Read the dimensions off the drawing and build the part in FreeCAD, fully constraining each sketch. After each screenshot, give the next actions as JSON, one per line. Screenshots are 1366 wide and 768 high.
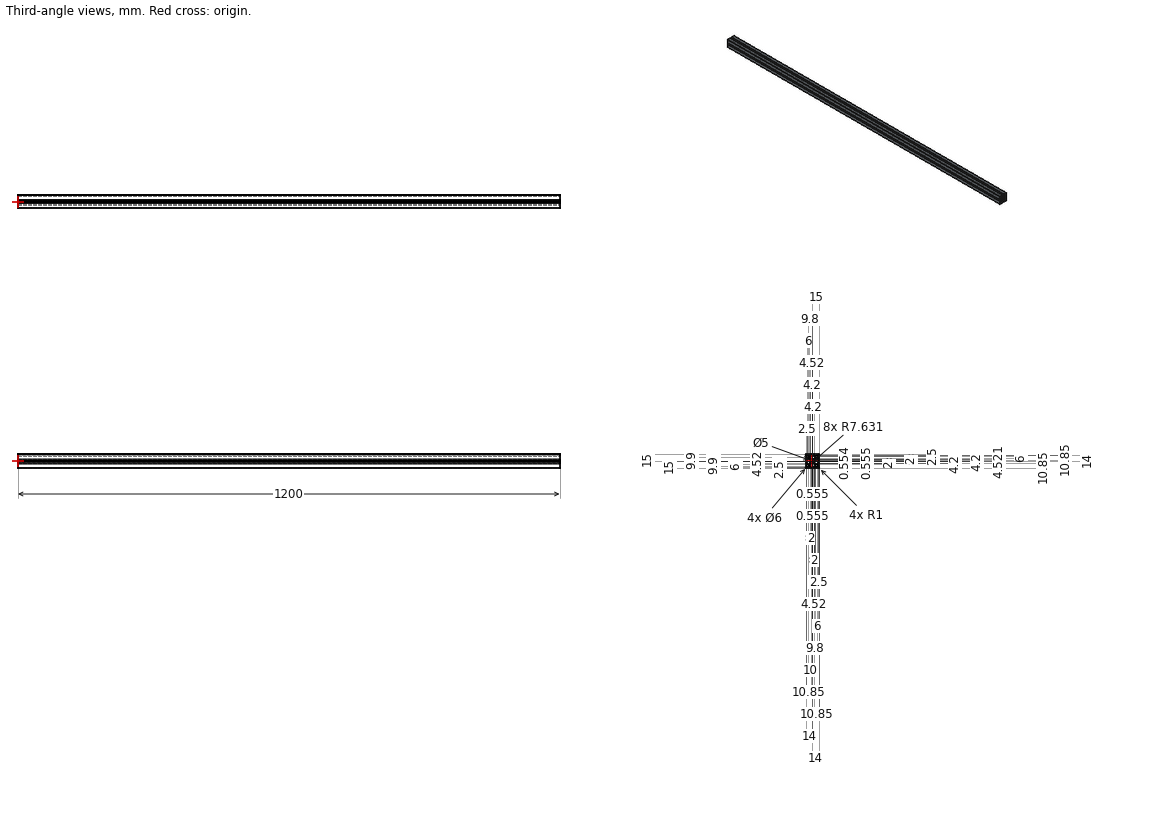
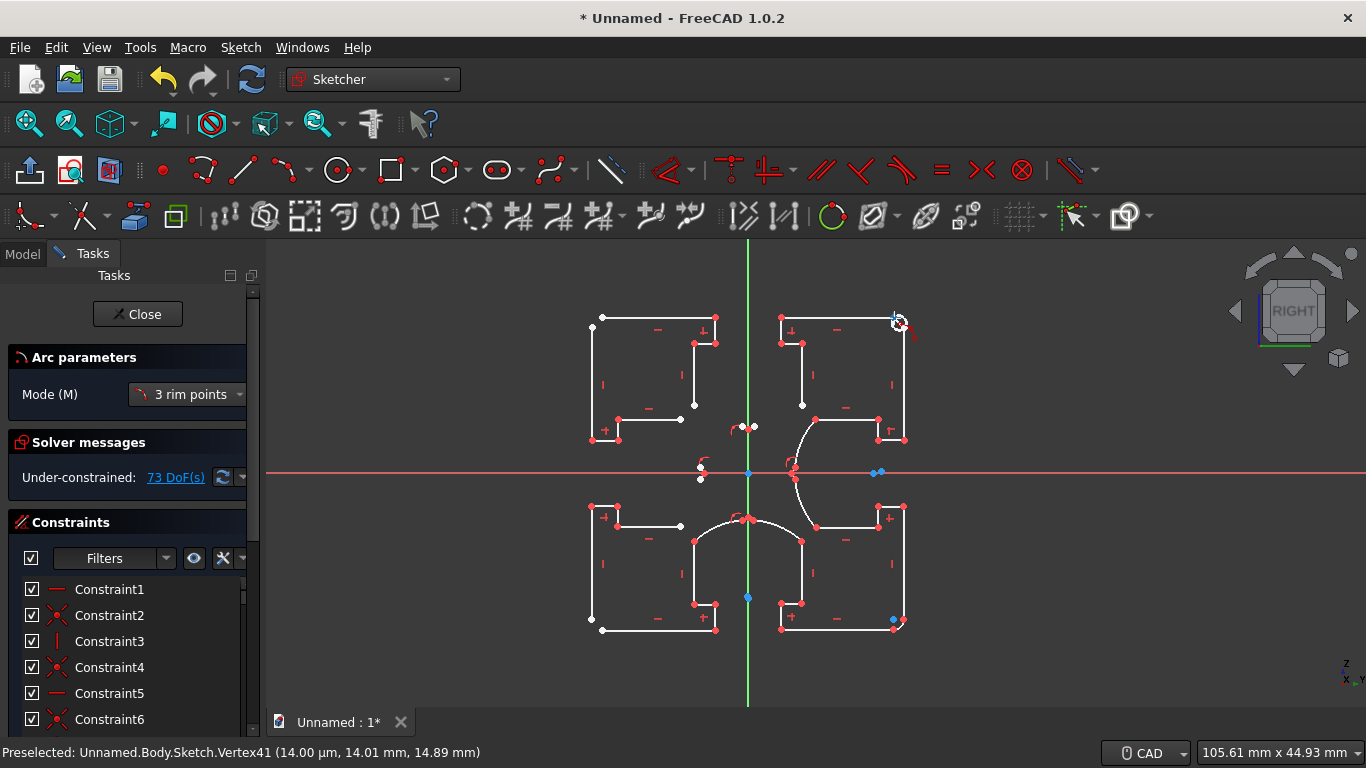
{"action": "scroll", "coordinate": [901, 320], "scroll_direction": "up", "scroll_amount": 9}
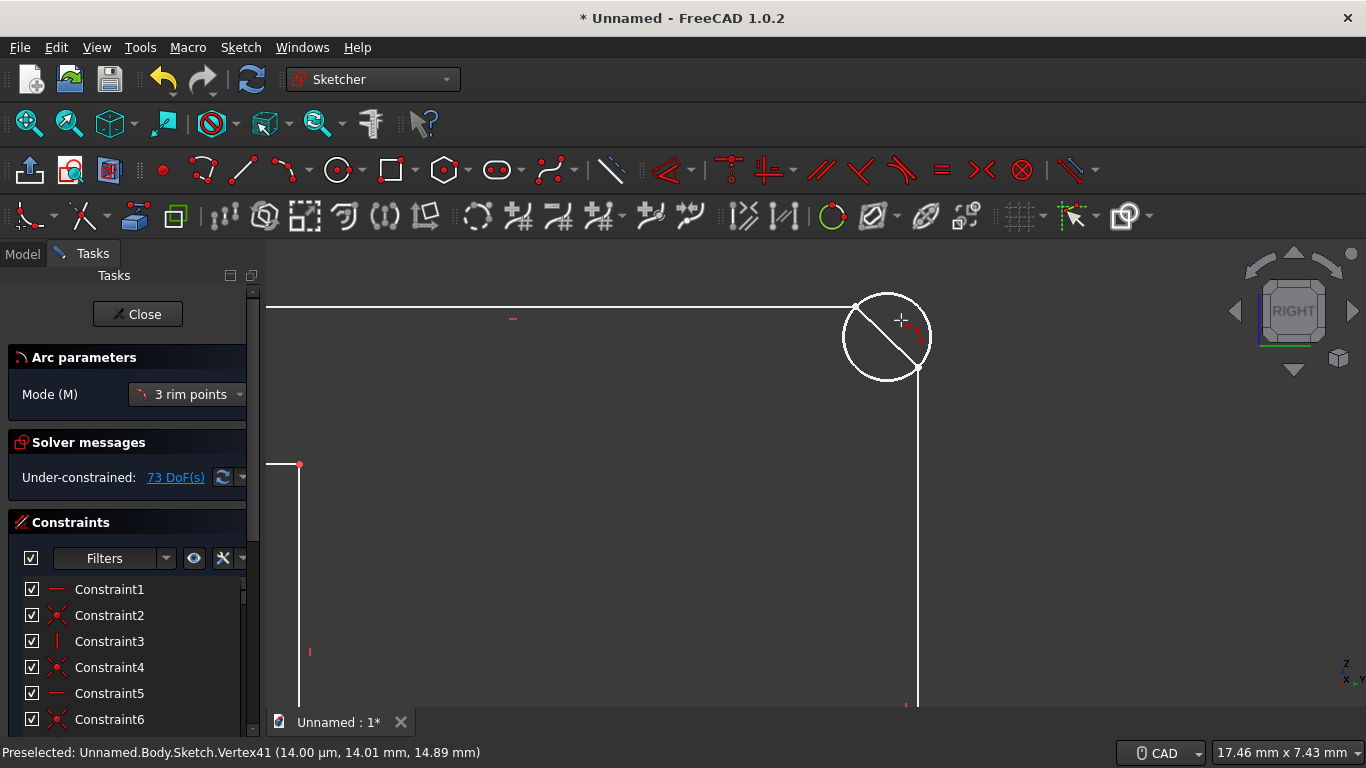
{"action": "left_click", "coordinate": [900, 318]}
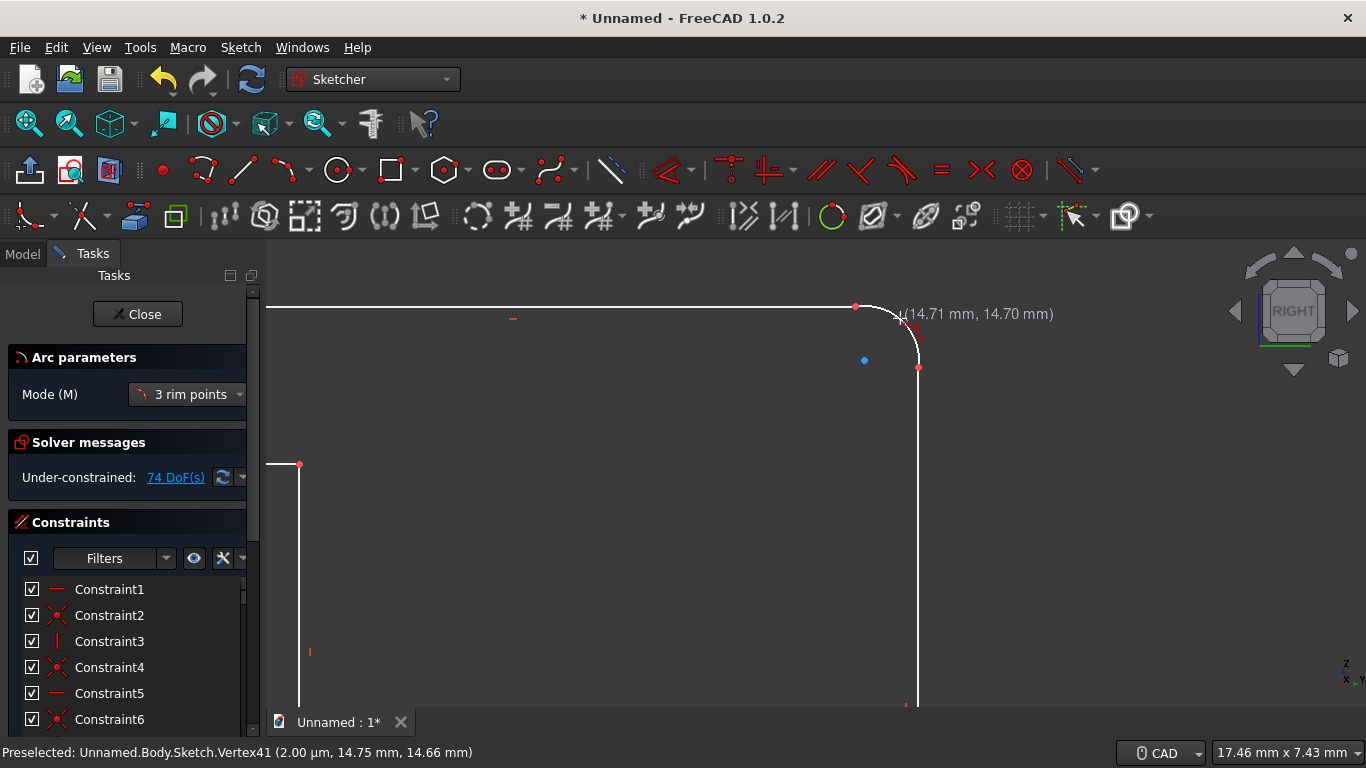
{"action": "scroll", "coordinate": [901, 320], "scroll_direction": "down", "scroll_amount": 9}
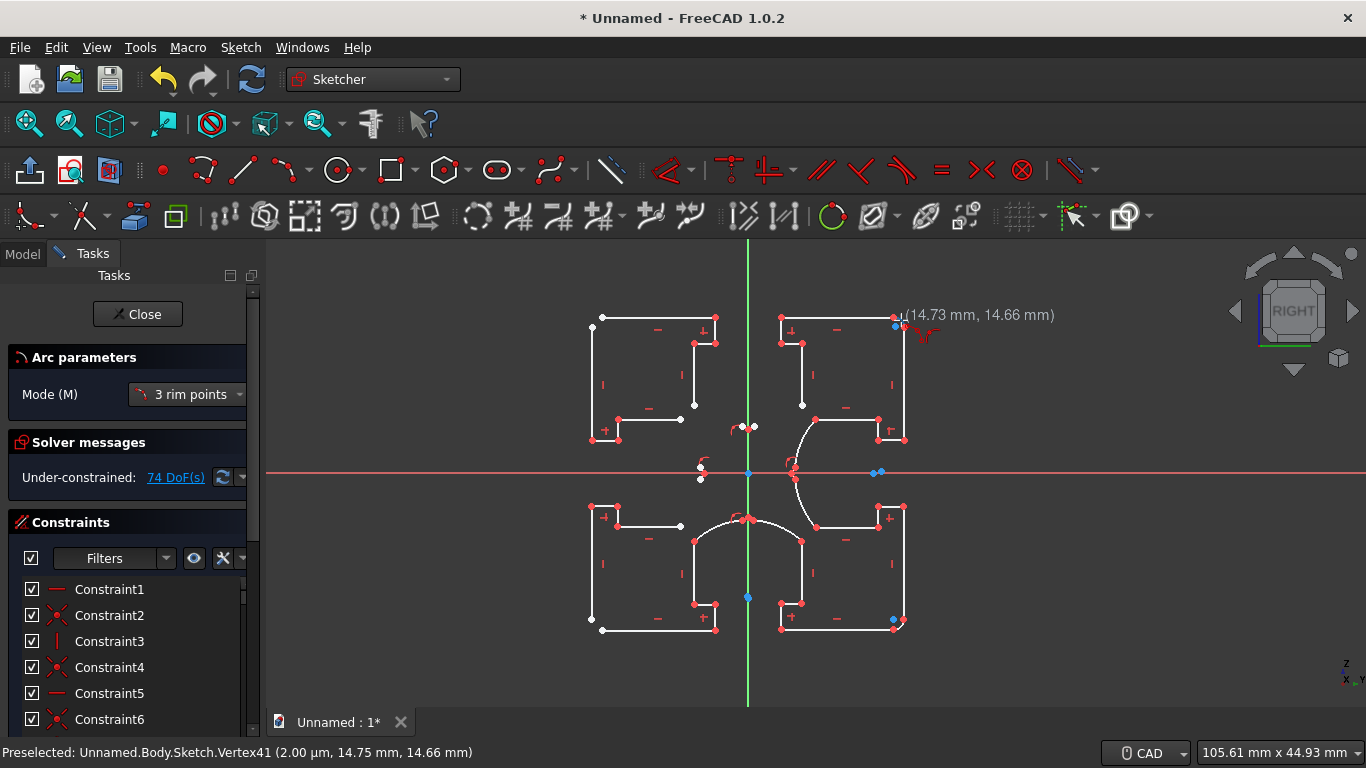
{"action": "left_click", "coordinate": [802, 406]}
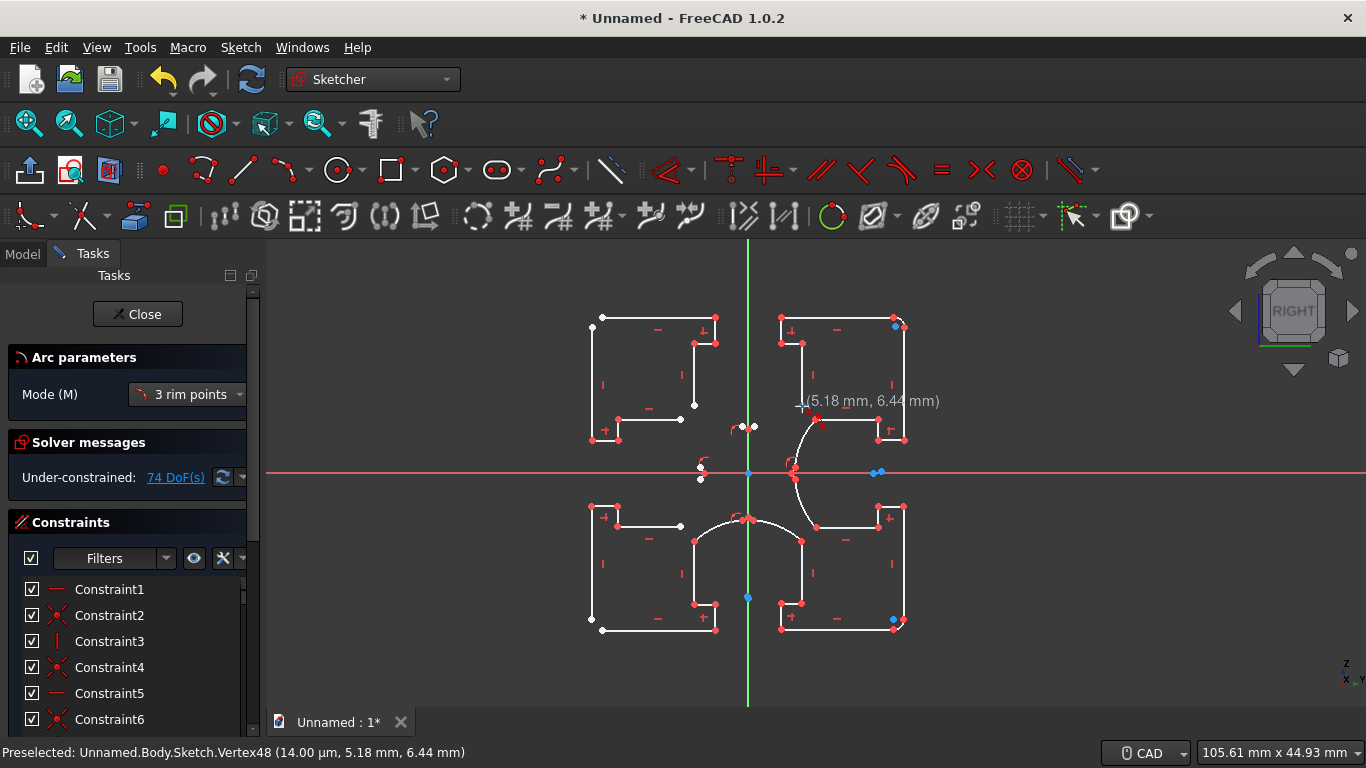
{"action": "scroll", "coordinate": [754, 426], "scroll_direction": "up", "scroll_amount": 8}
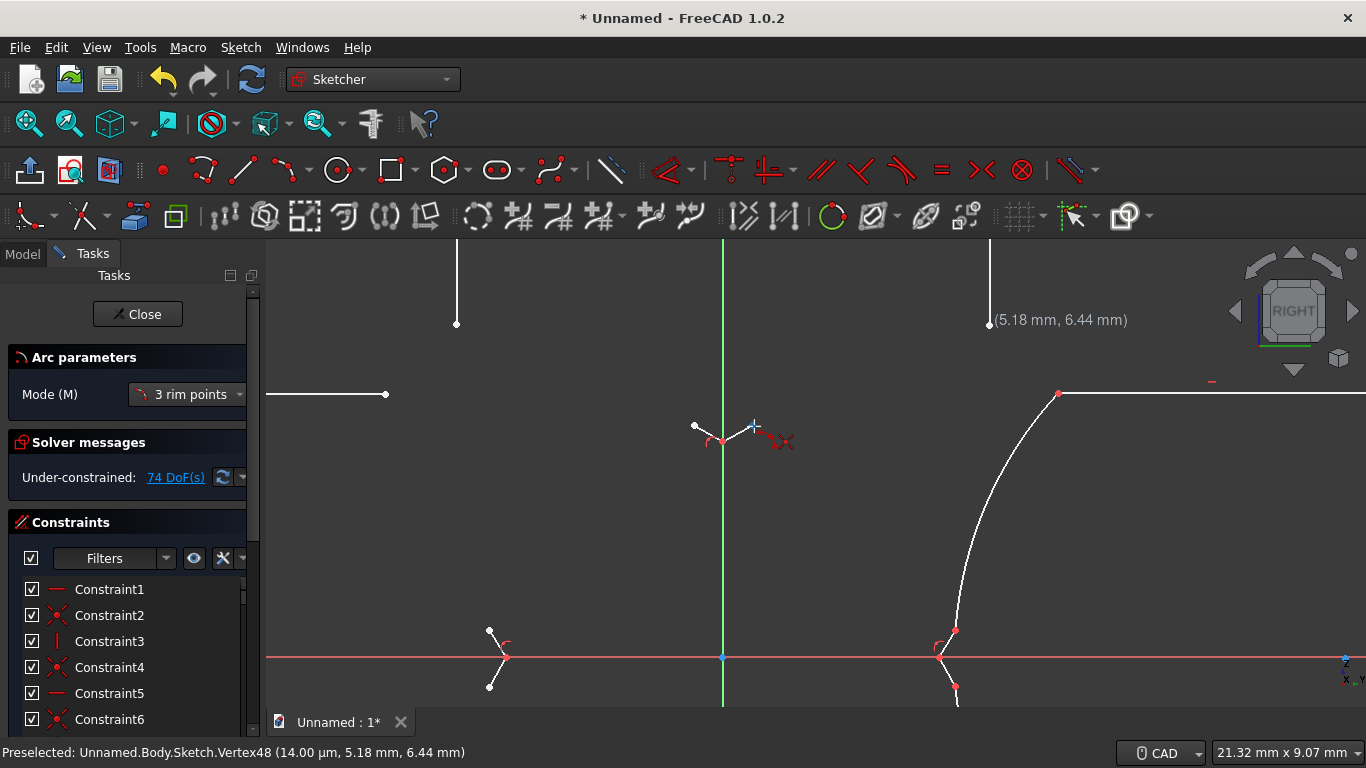
{"action": "left_click", "coordinate": [752, 426]}
{"action": "left_click", "coordinate": [879, 393]}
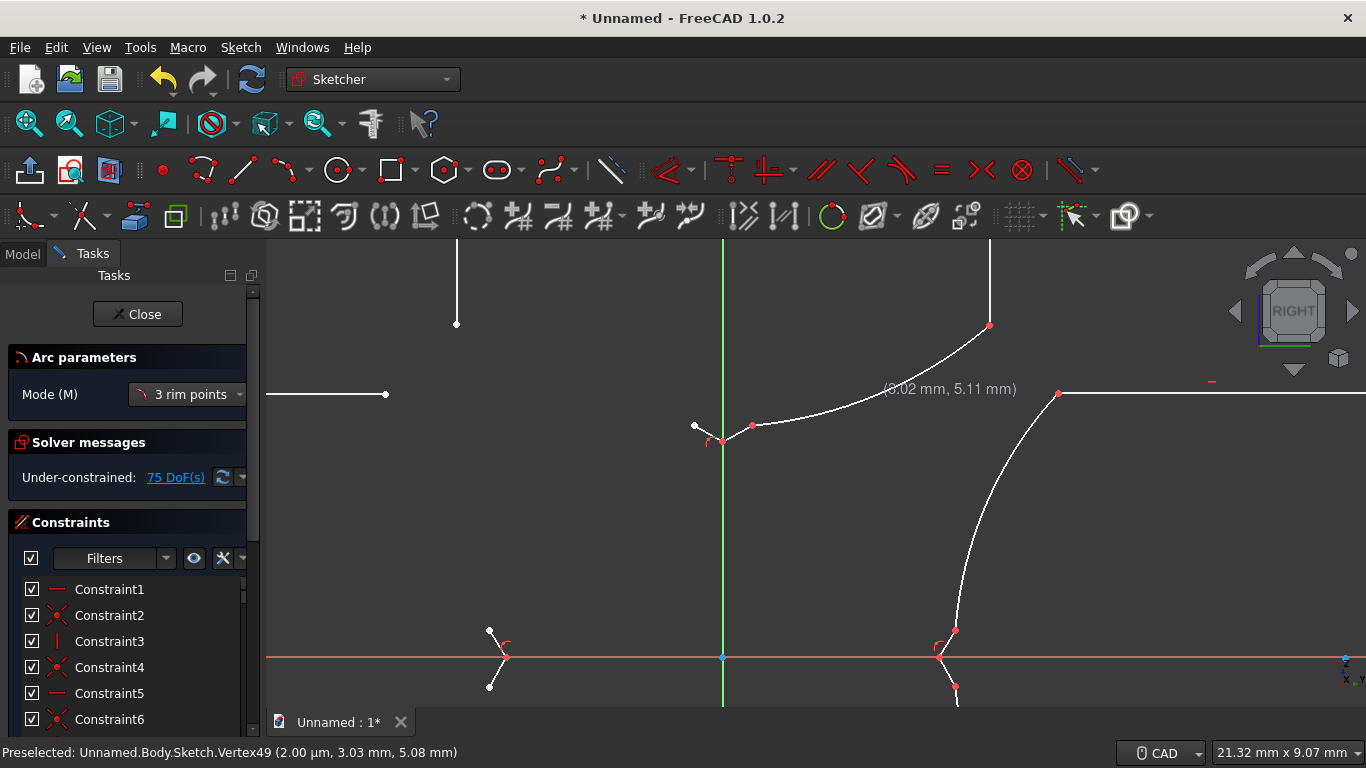
{"action": "left_click", "coordinate": [694, 426]}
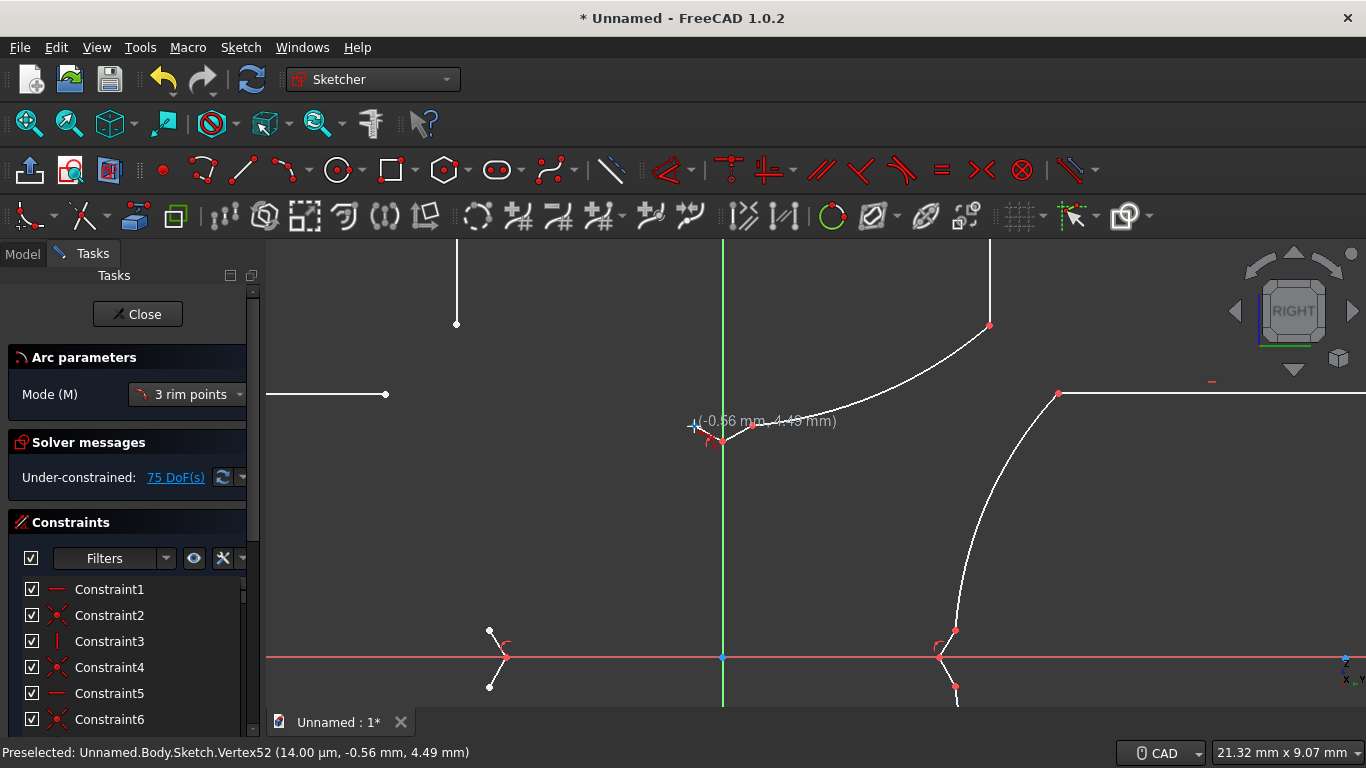
{"action": "scroll", "coordinate": [754, 426], "scroll_direction": "down", "scroll_amount": 8}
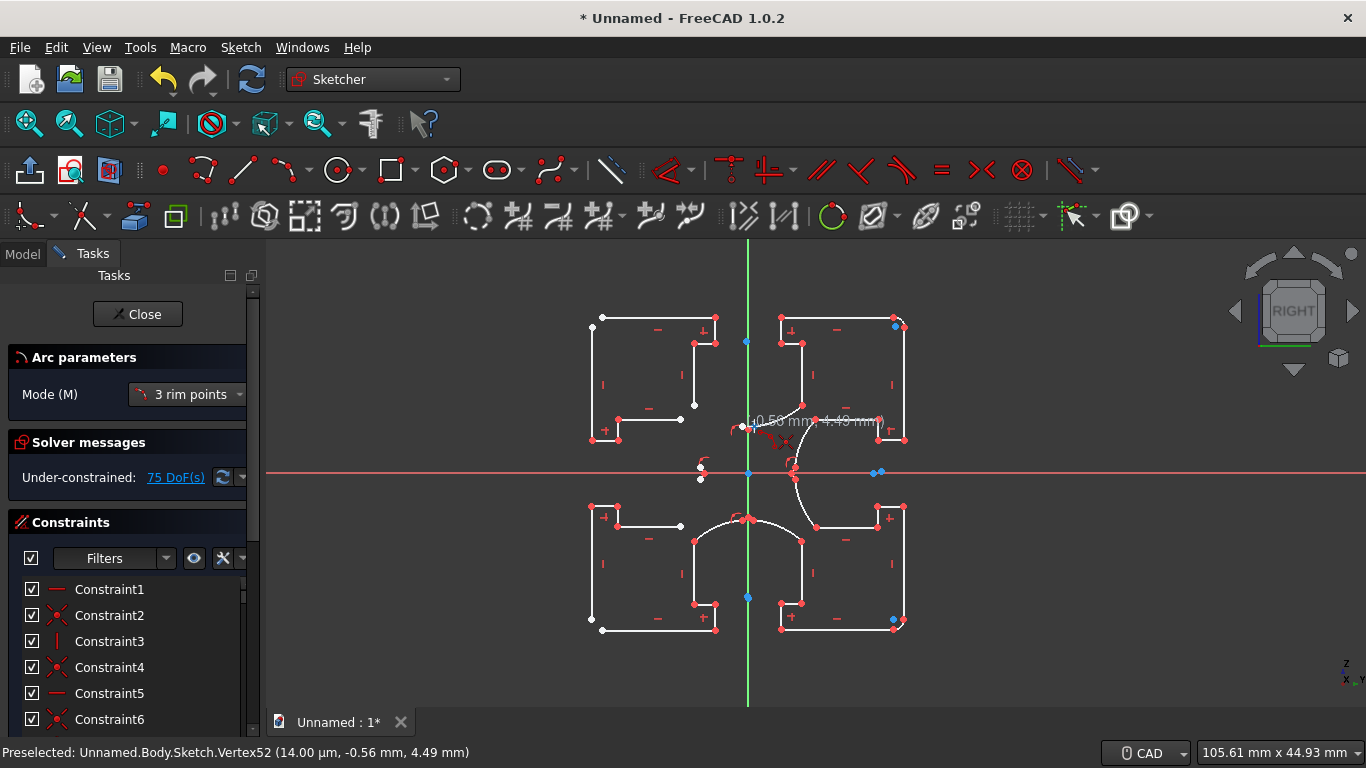
{"action": "left_click", "coordinate": [694, 406]}